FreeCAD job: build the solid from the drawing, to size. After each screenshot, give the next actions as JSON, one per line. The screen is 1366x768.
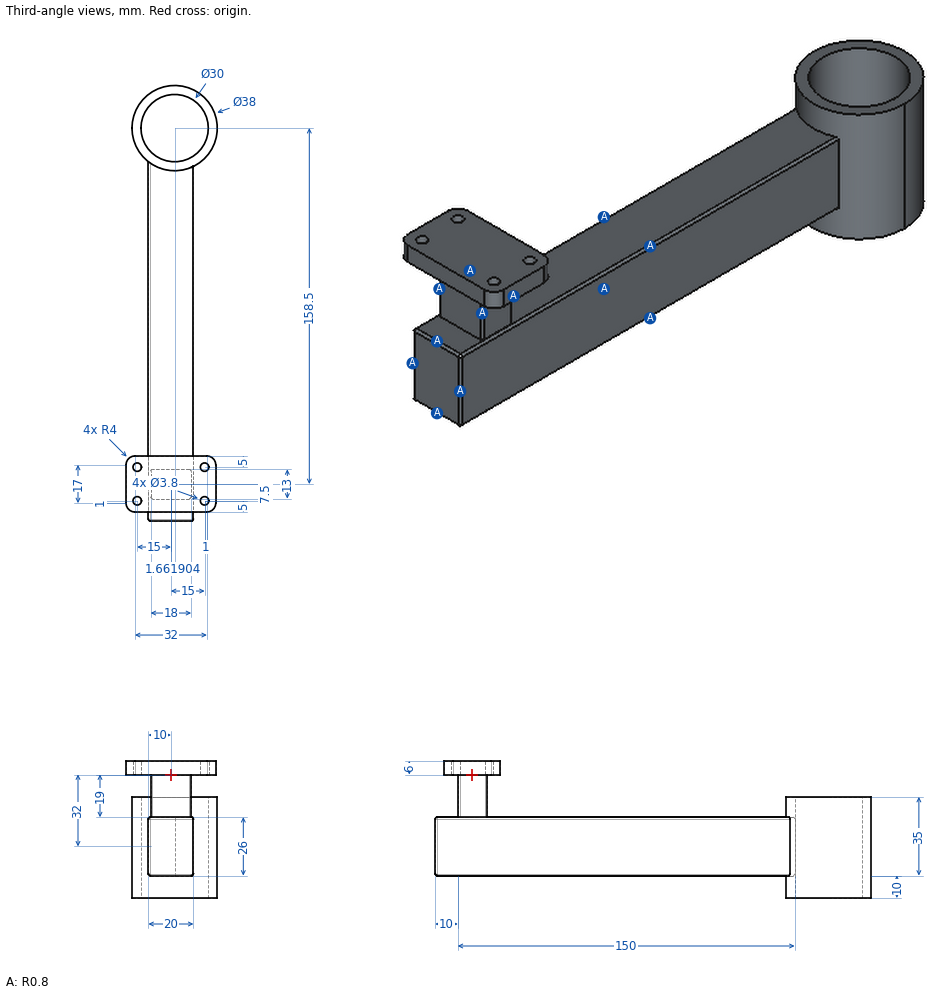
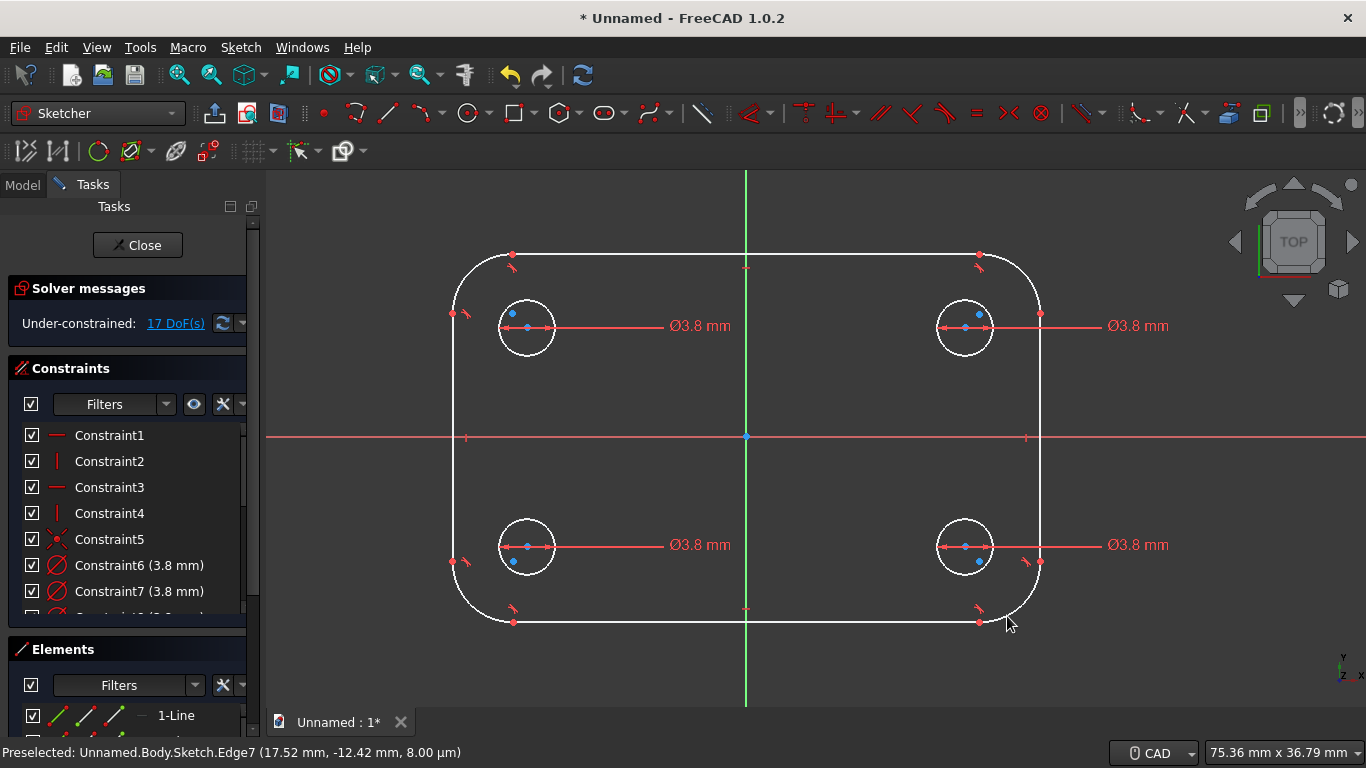
{"action": "left_click", "coordinate": [1040, 488]}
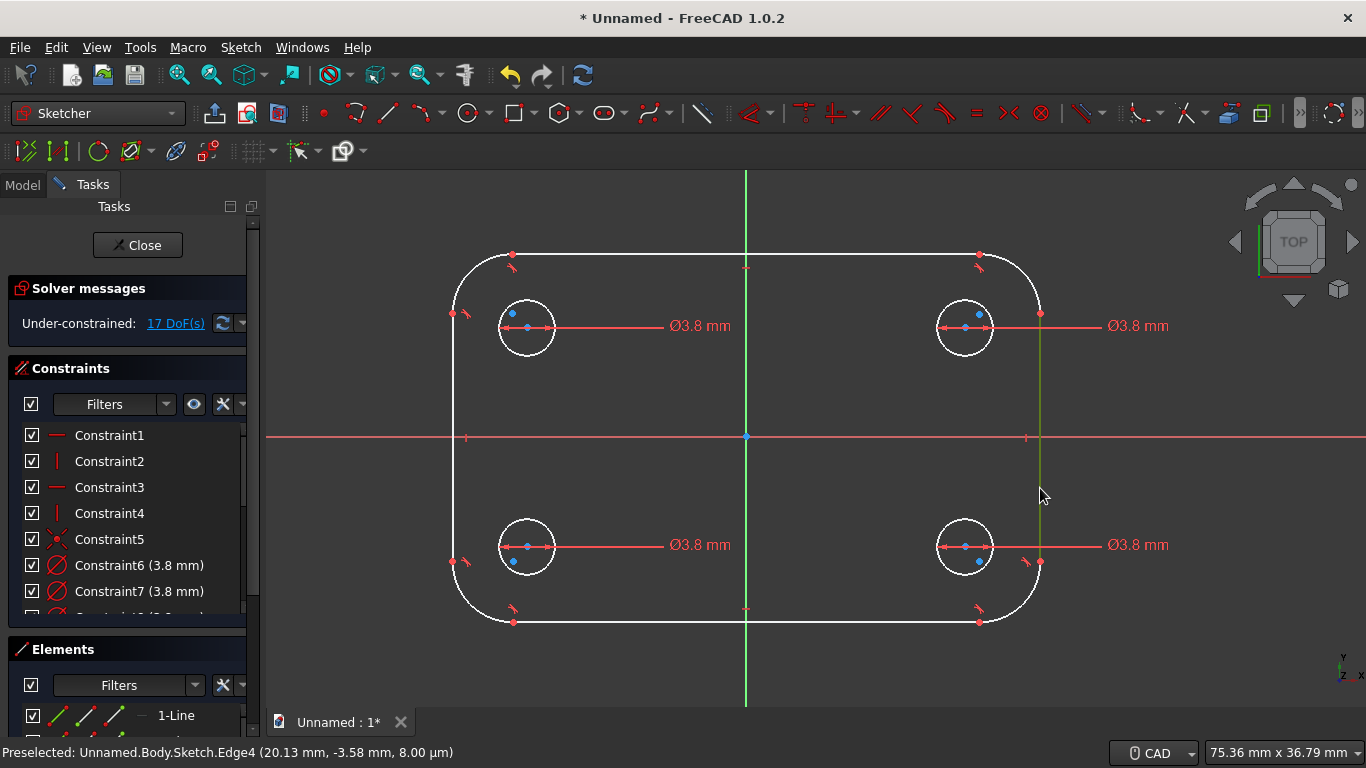
{"action": "left_click", "coordinate": [1033, 287]}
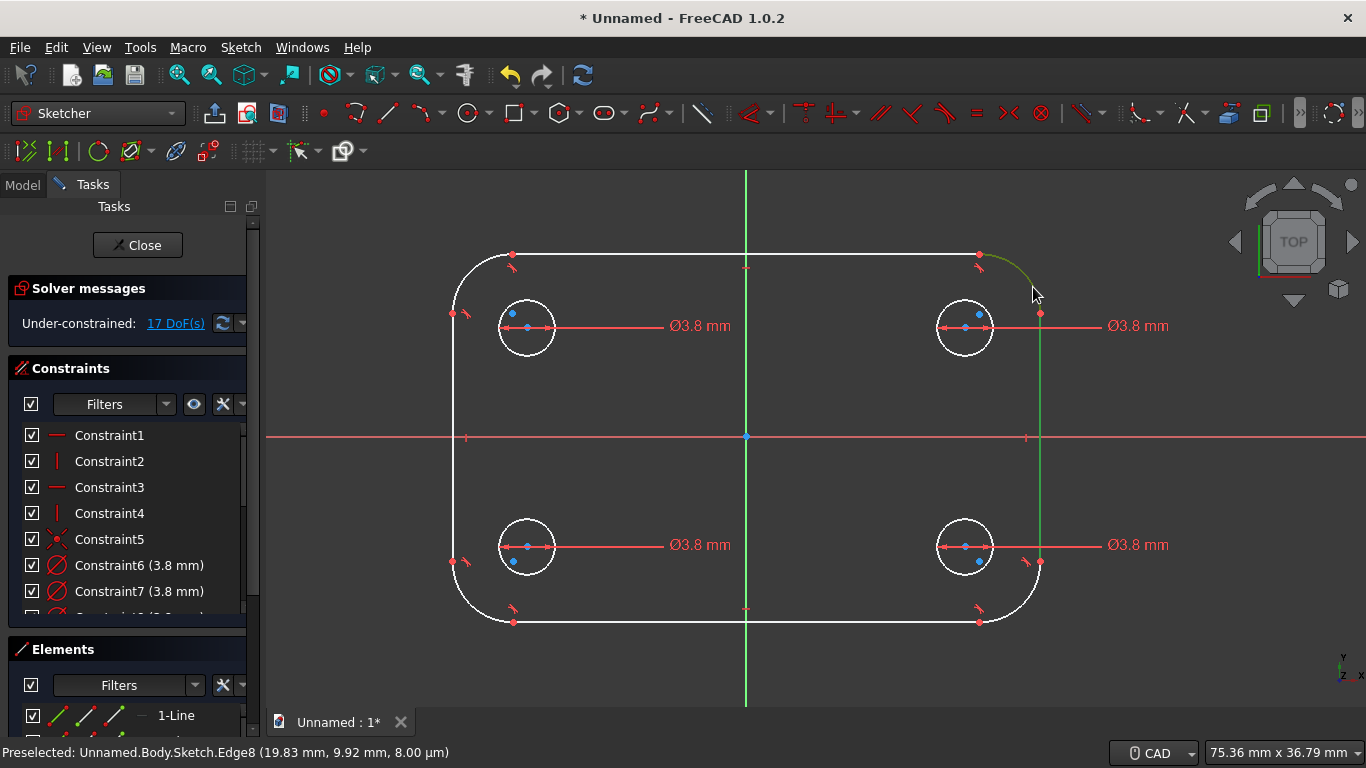
{"action": "left_click", "coordinate": [946, 114]}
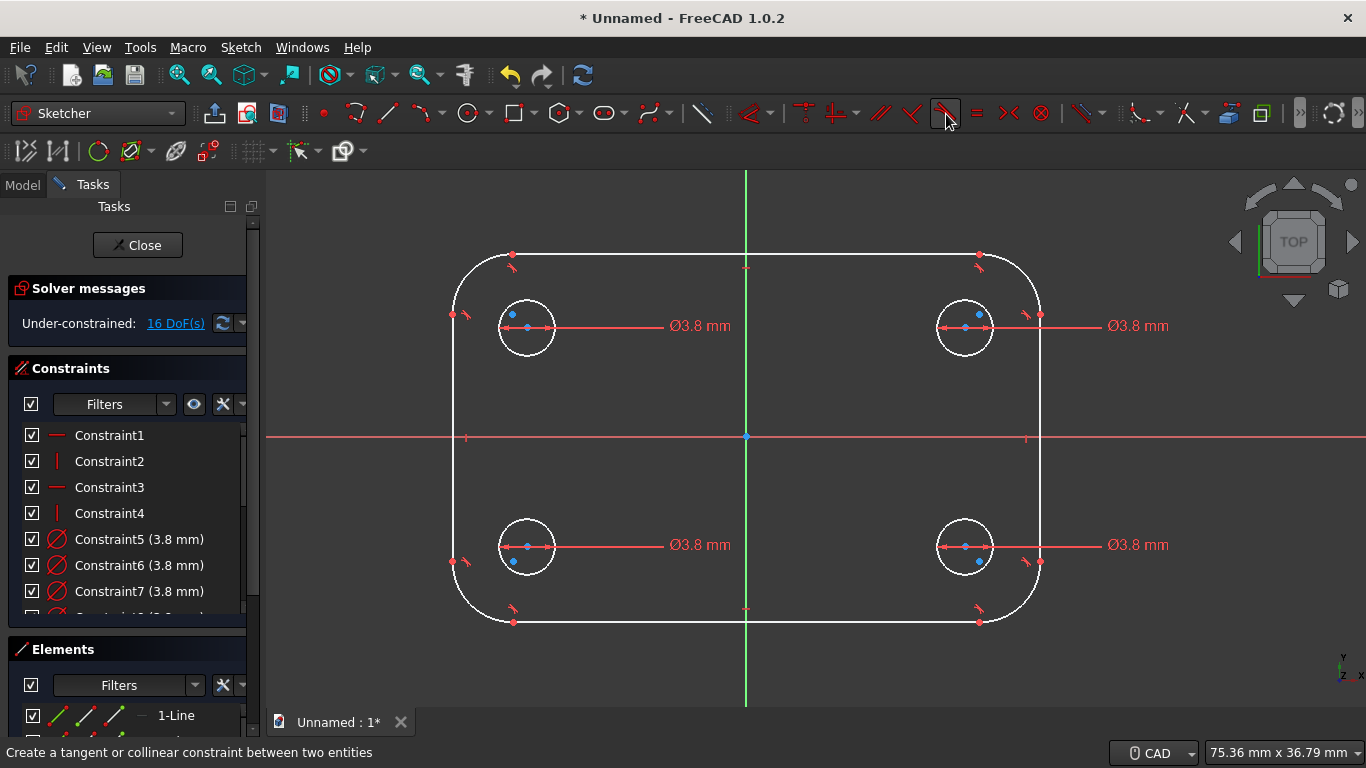
{"action": "left_click", "coordinate": [485, 261]}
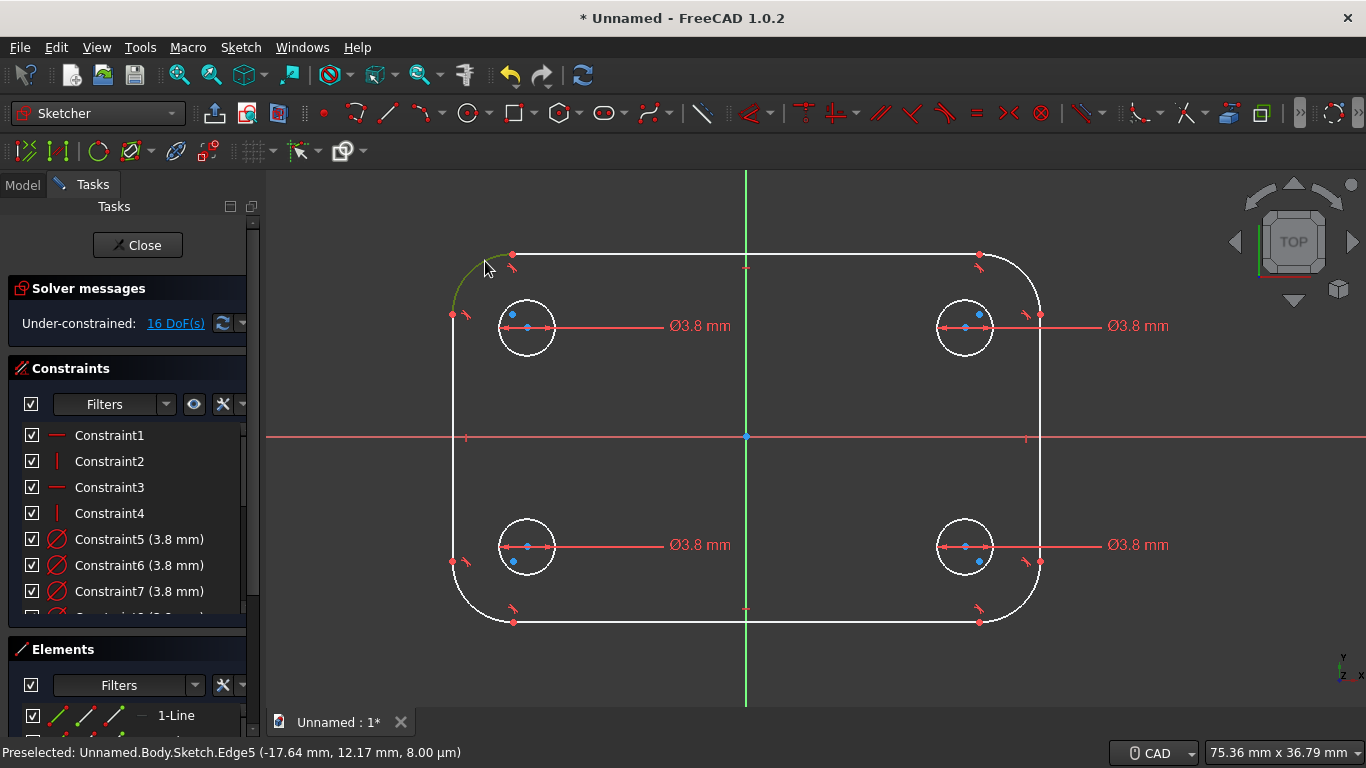
{"action": "left_click", "coordinate": [459, 589]}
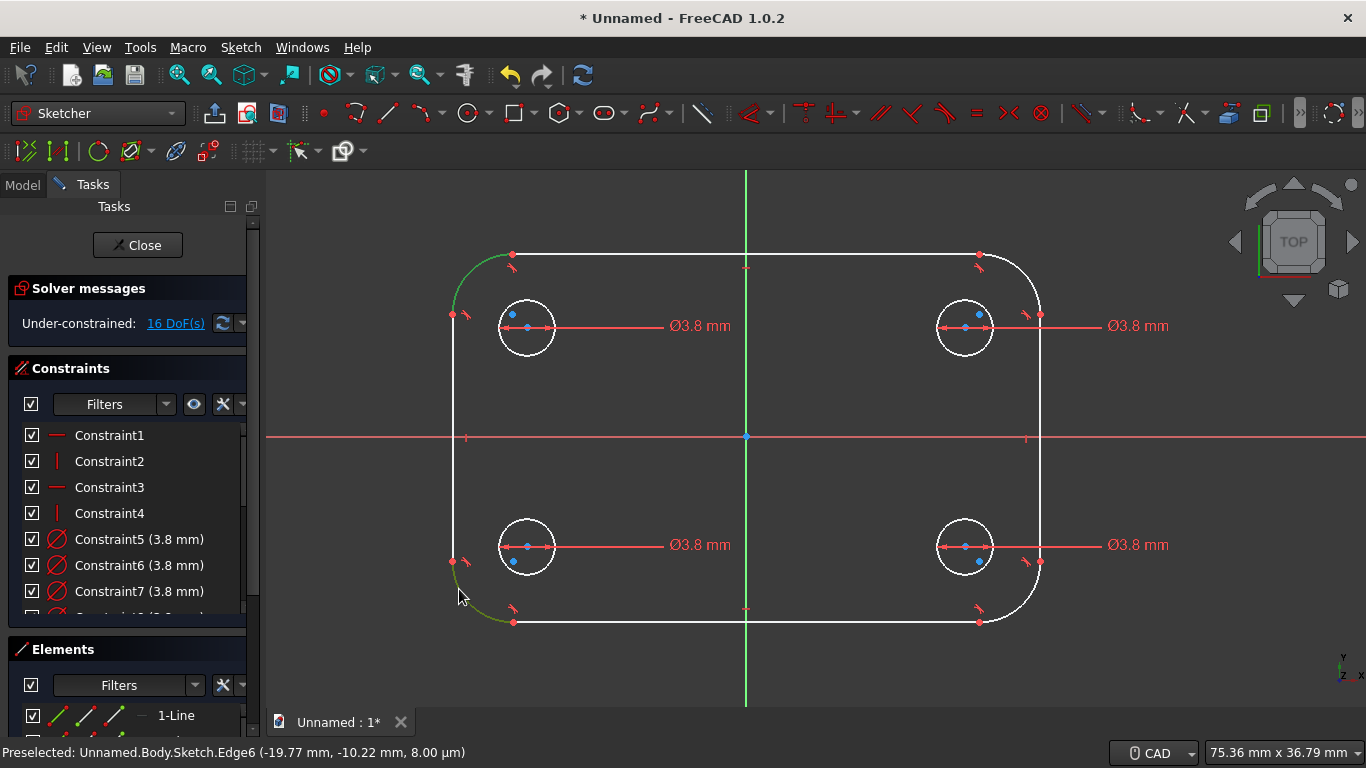
{"action": "left_click", "coordinate": [1007, 616]}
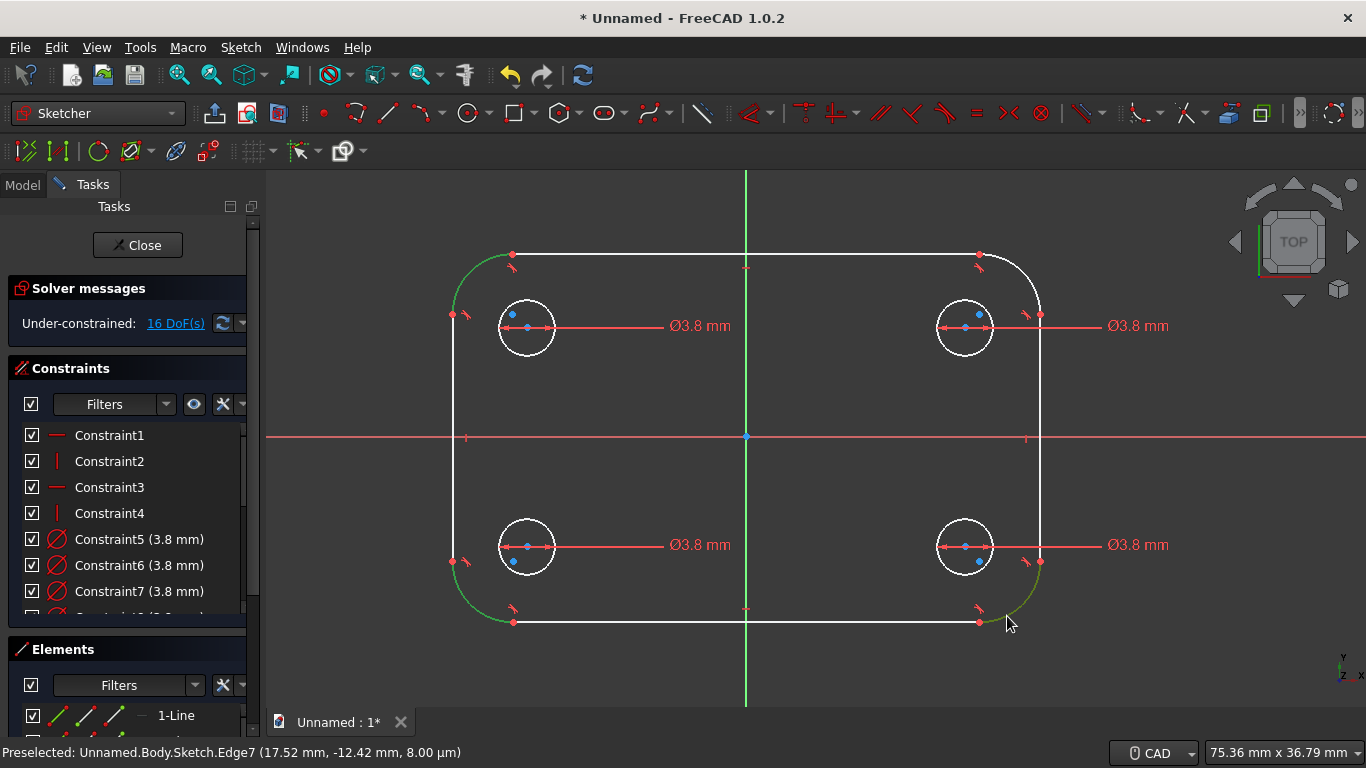
{"action": "left_click", "coordinate": [1034, 287]}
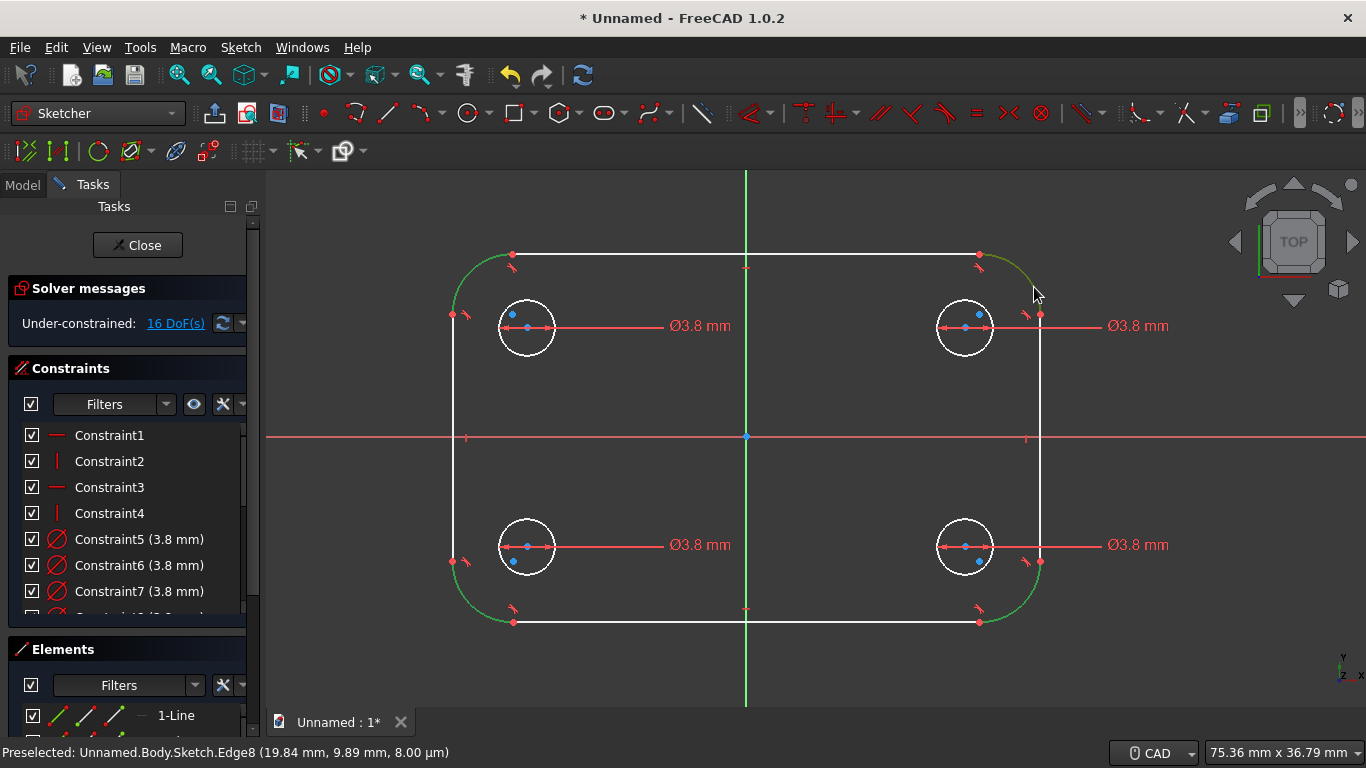
{"action": "left_click", "coordinate": [978, 114]}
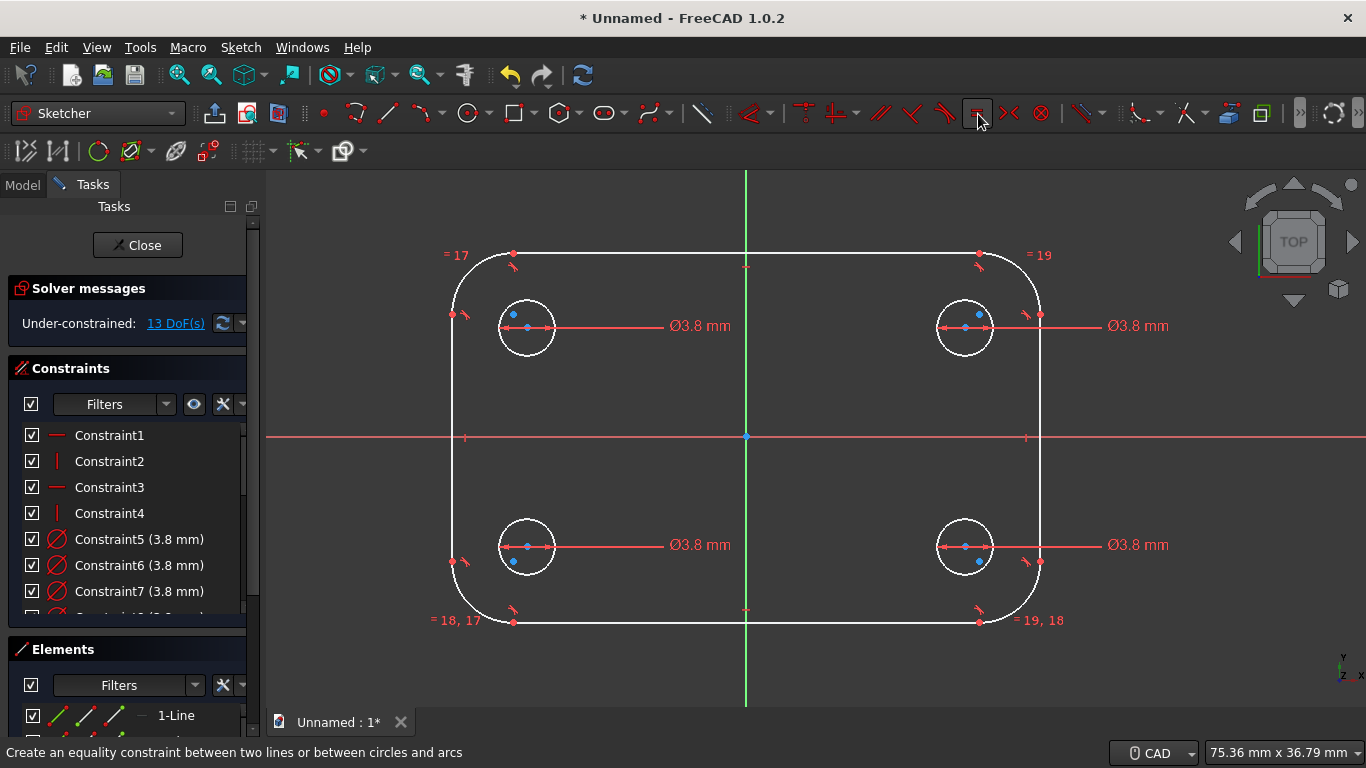
{"action": "left_click", "coordinate": [965, 547]}